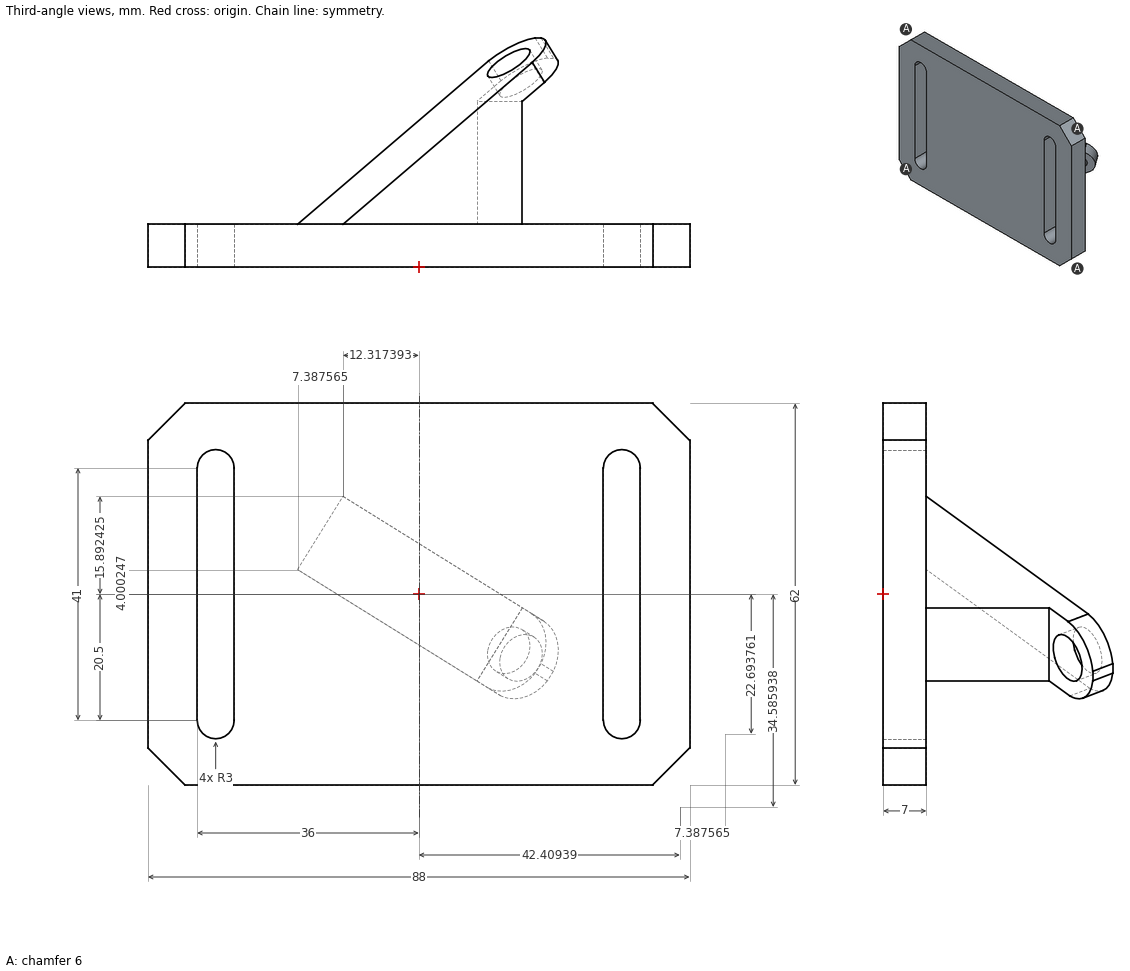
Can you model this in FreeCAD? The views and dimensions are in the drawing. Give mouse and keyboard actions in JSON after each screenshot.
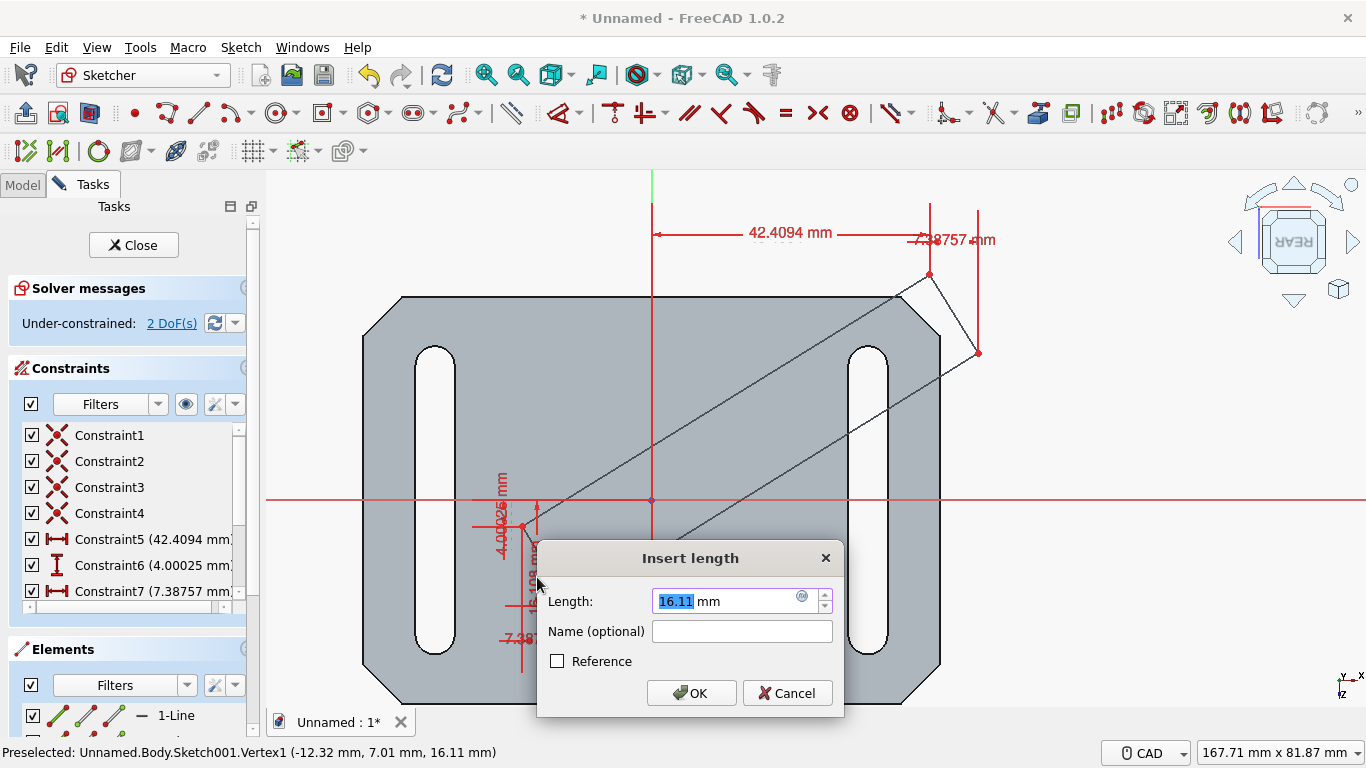
{"action": "type", "text": "15.892425"}
{"action": "key", "text": "Return"}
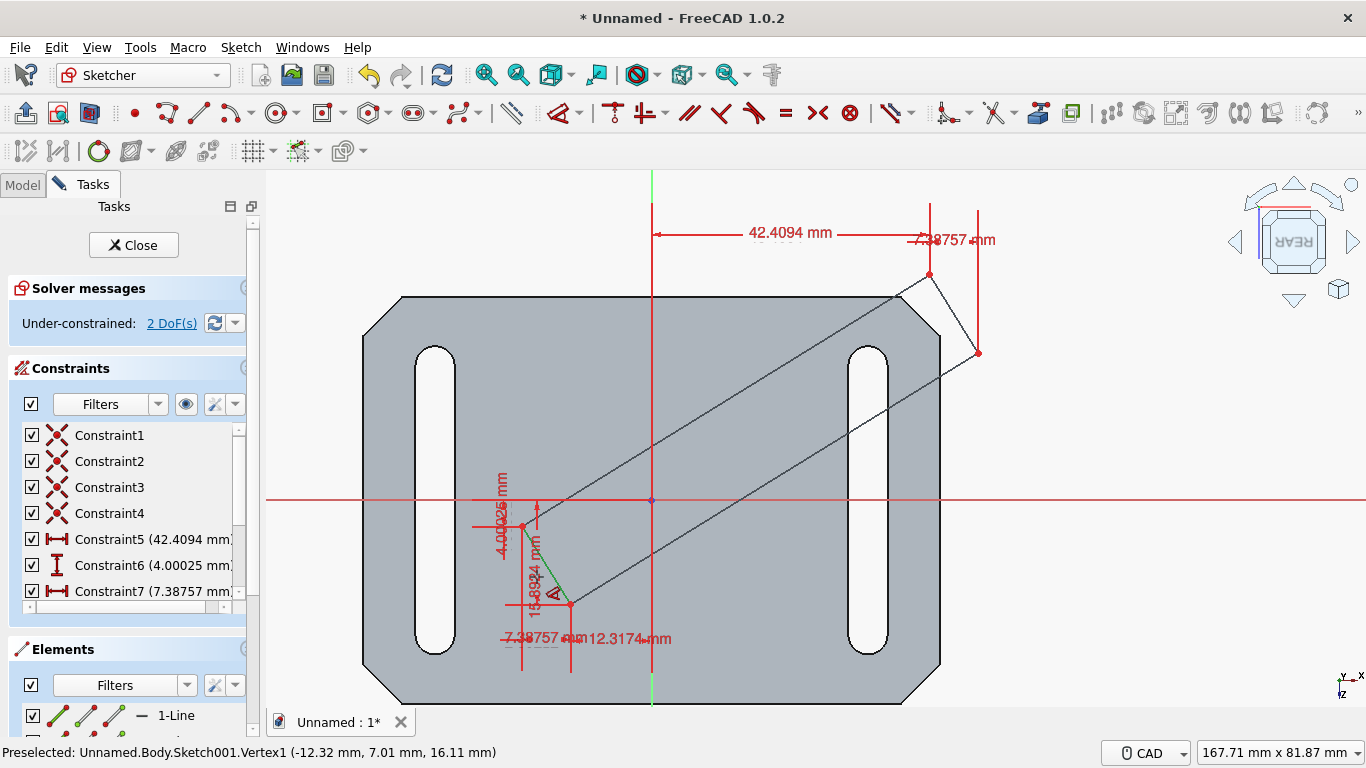
{"action": "left_click", "coordinate": [978, 353]}
{"action": "left_click", "coordinate": [1012, 427]}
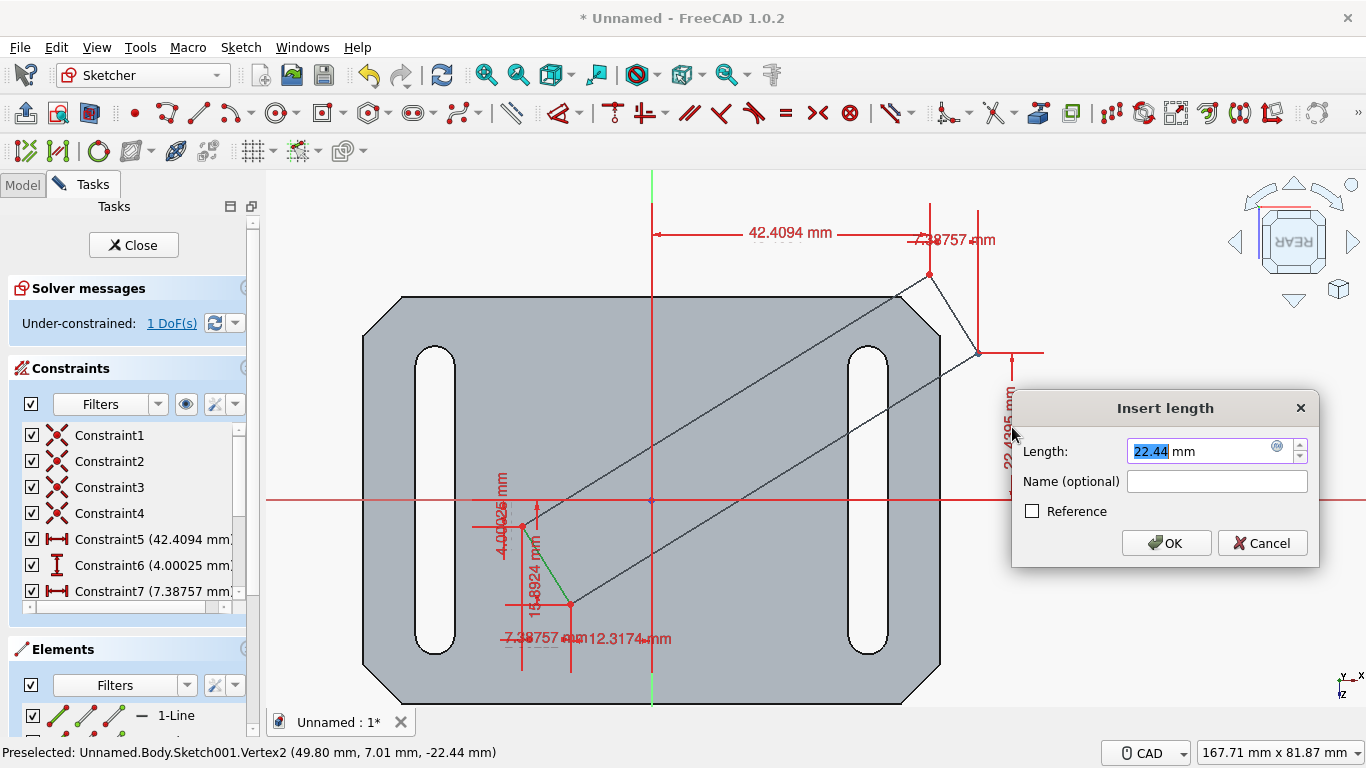
{"action": "type", "text": "22.693761"}
{"action": "key", "text": "Return"}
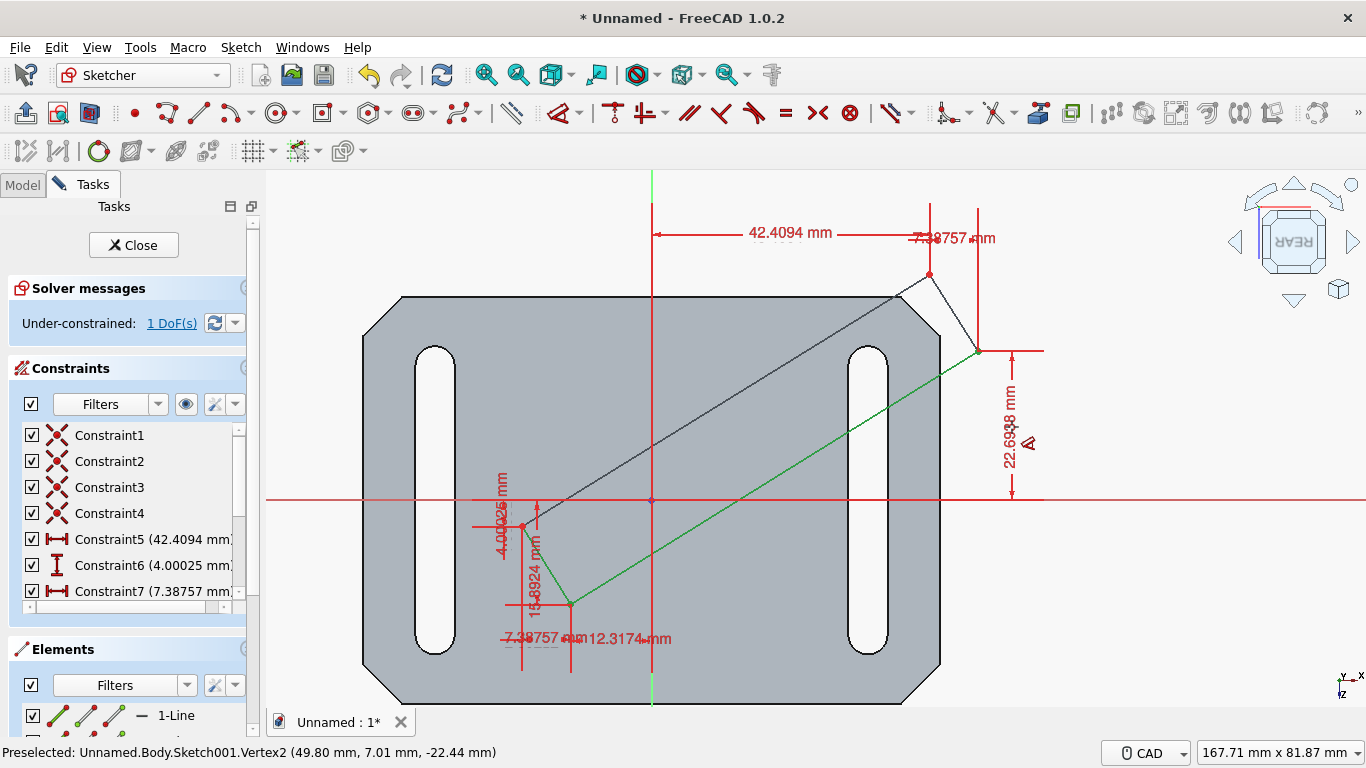
{"action": "left_click", "coordinate": [930, 275]}
{"action": "left_click", "coordinate": [964, 388]}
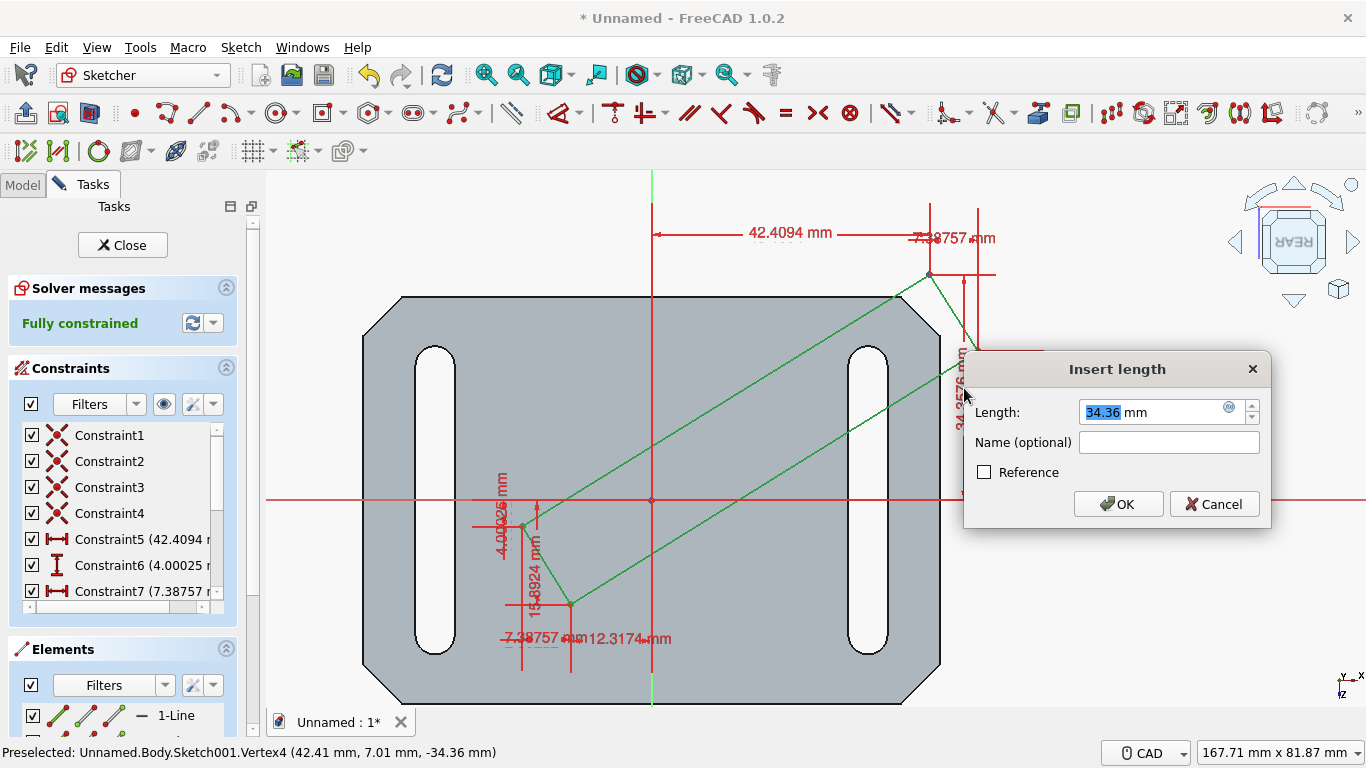
{"action": "type", "text": "34.585938"}
{"action": "key", "text": "Return"}
{"action": "key", "text": "Escape"}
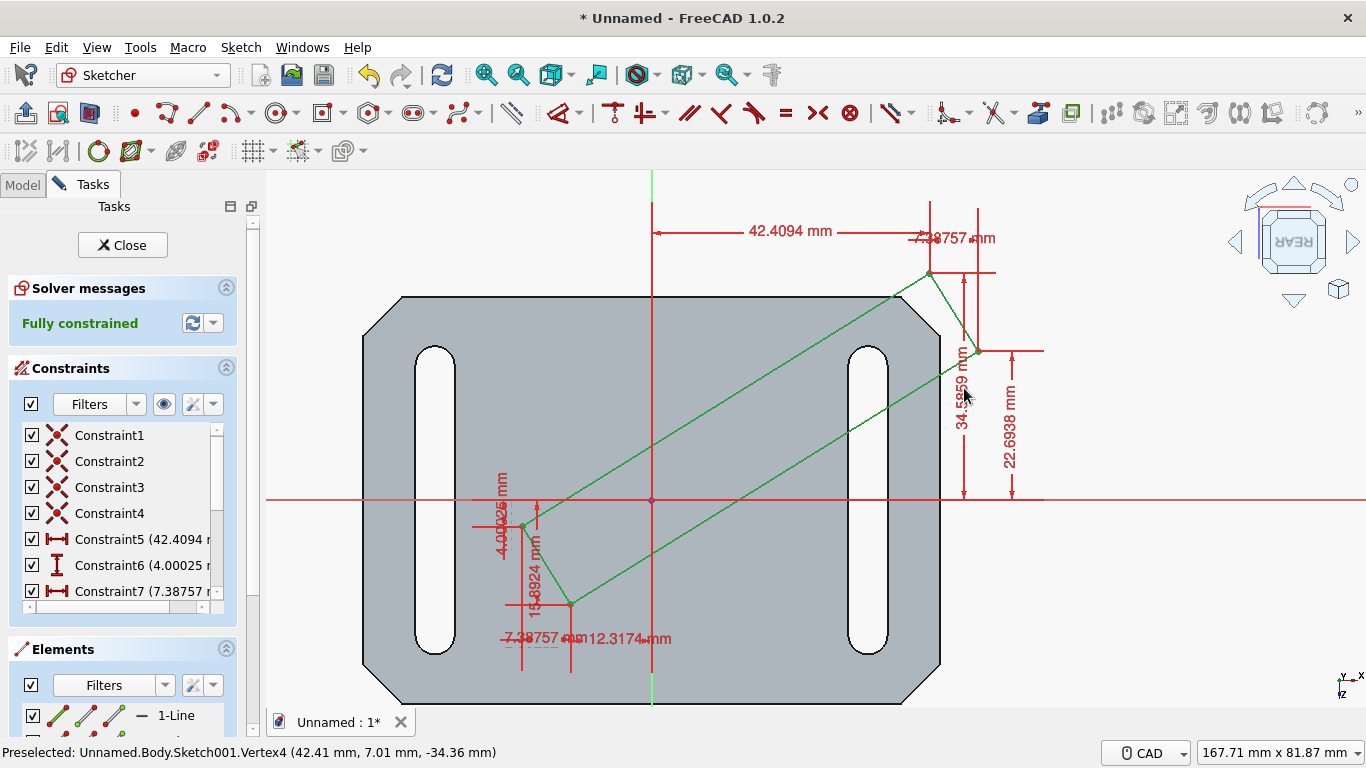
{"action": "left_click", "coordinate": [123, 245]}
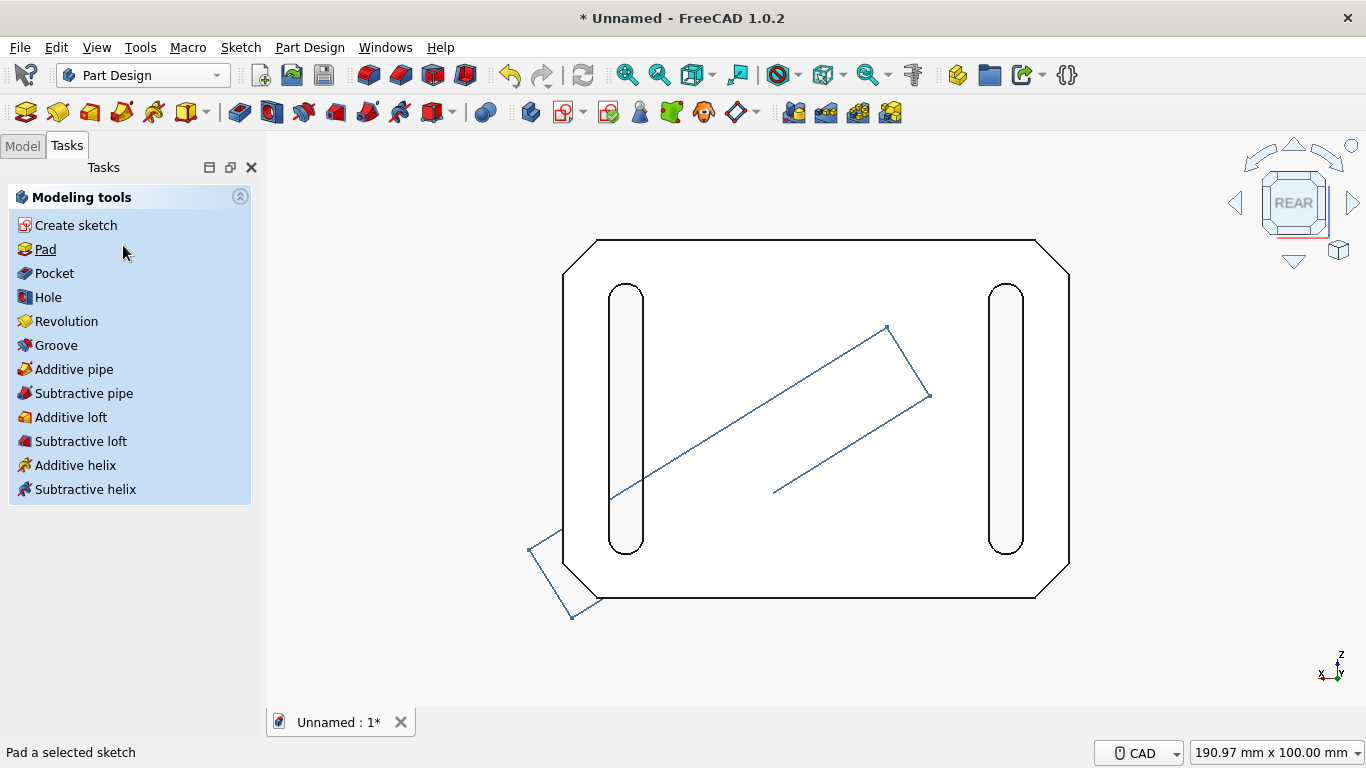
{"action": "left_click", "coordinate": [26, 112]}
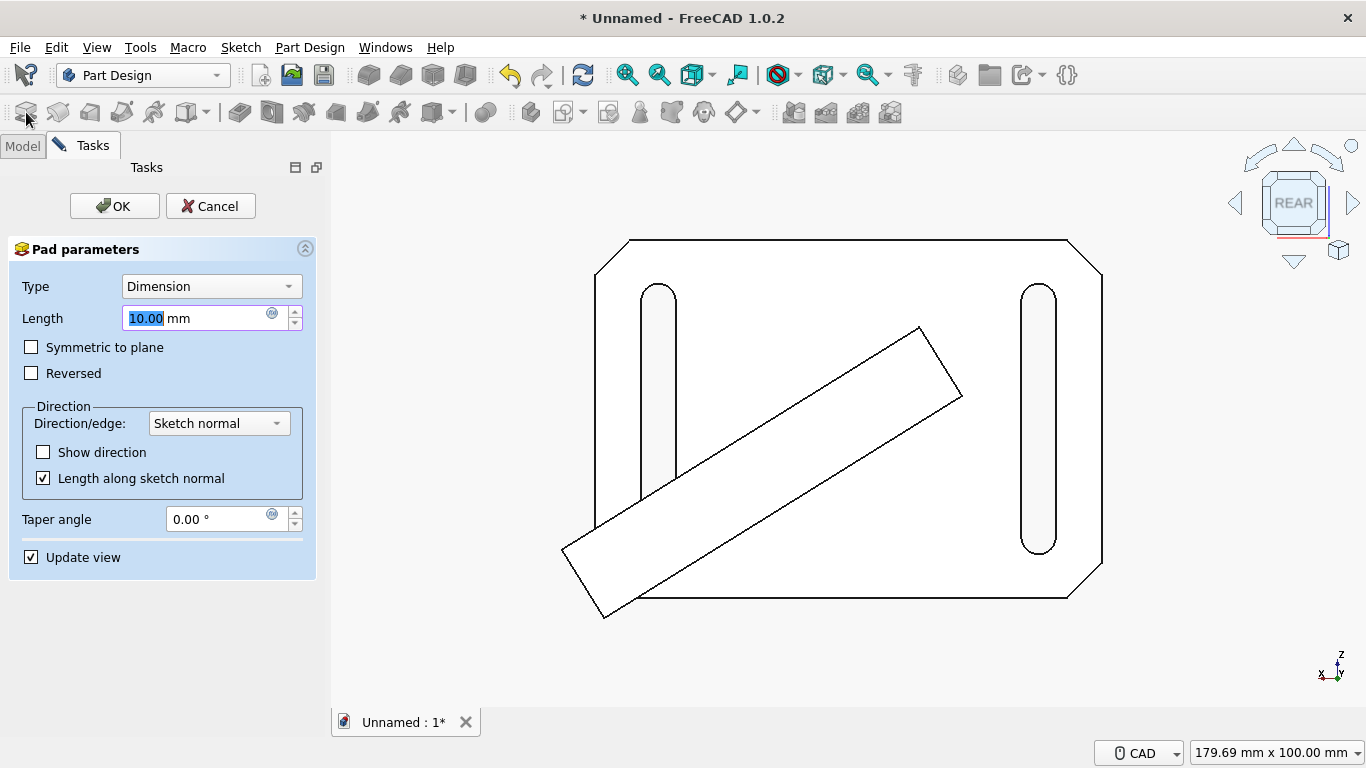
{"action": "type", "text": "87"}
{"action": "key", "text": "Tab"}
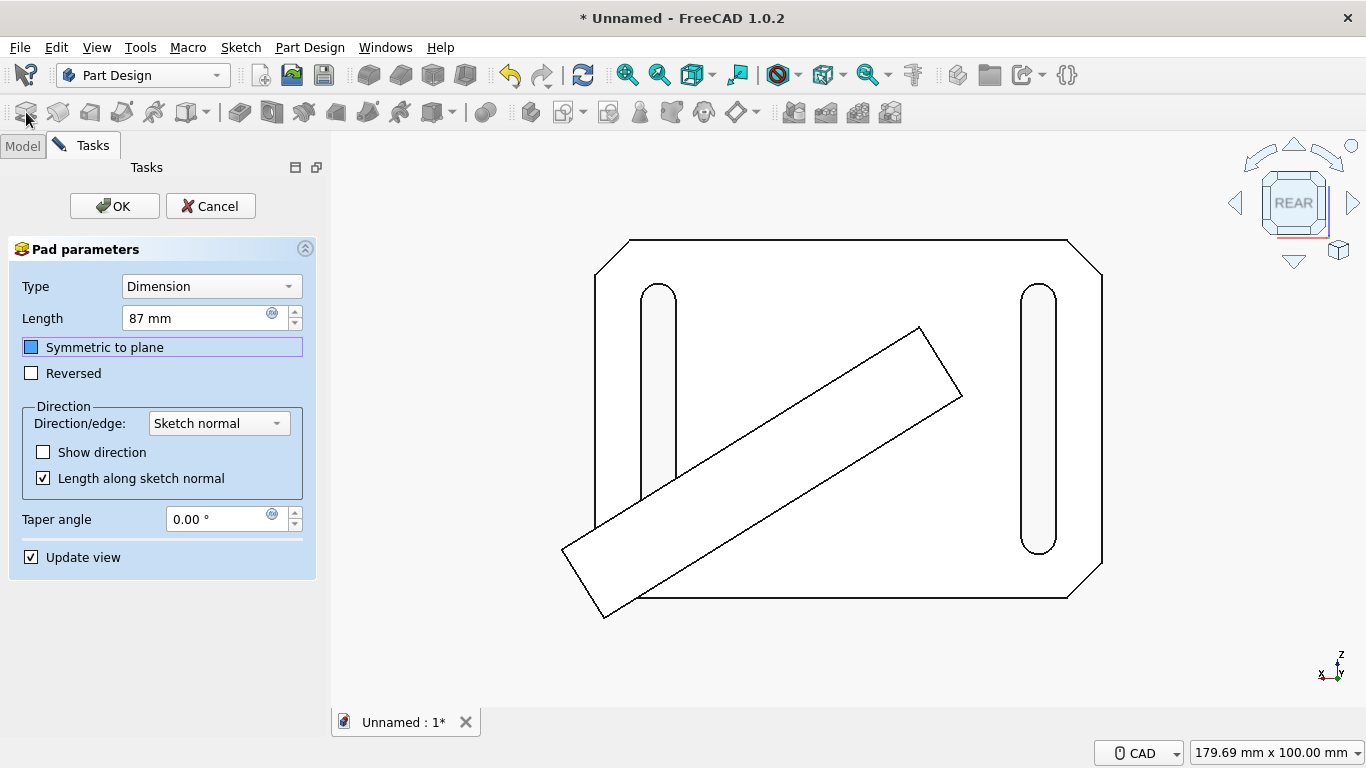
{"action": "left_click", "coordinate": [115, 206]}